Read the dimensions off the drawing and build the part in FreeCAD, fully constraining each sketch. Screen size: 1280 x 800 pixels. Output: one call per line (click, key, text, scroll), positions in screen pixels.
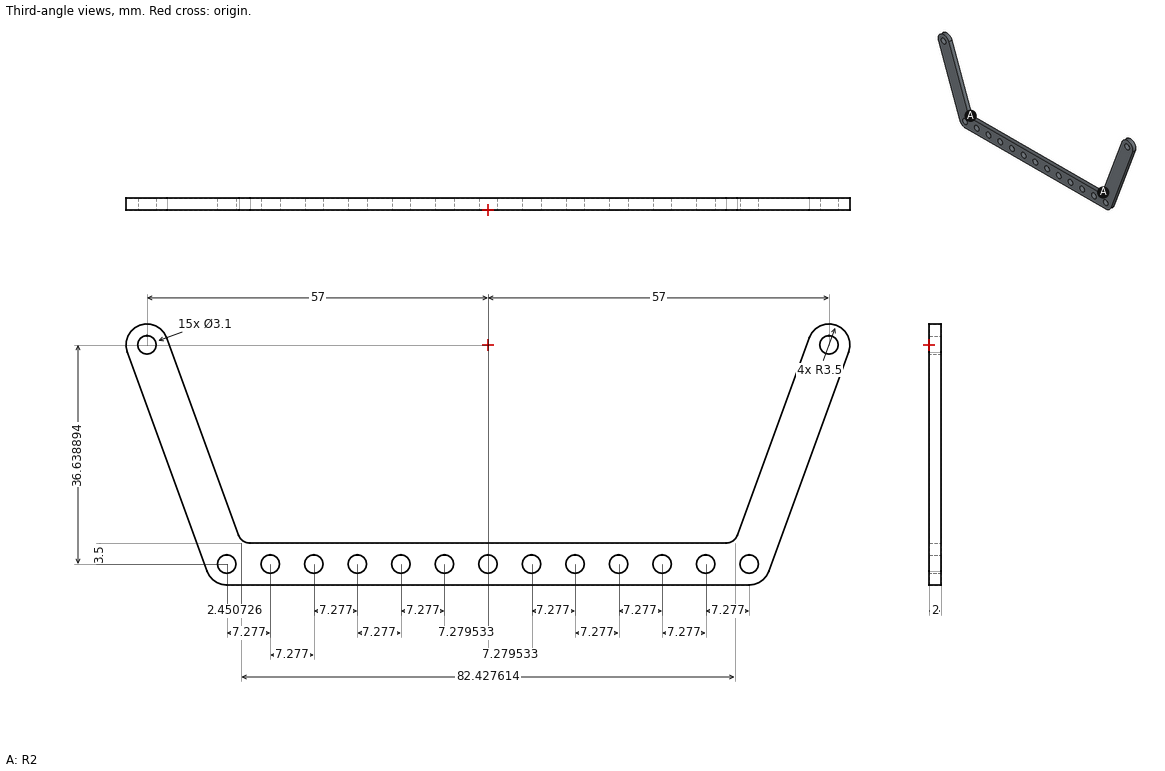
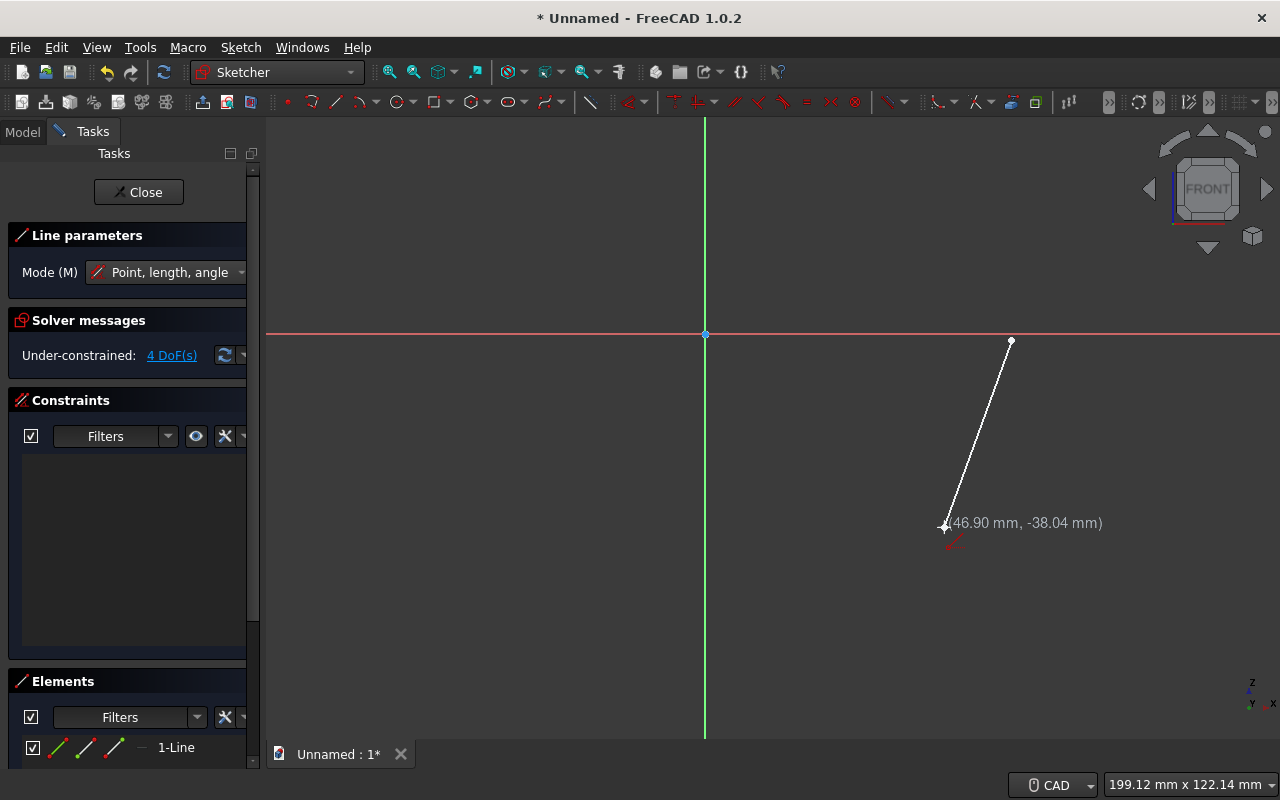
click(927, 539)
click(483, 539)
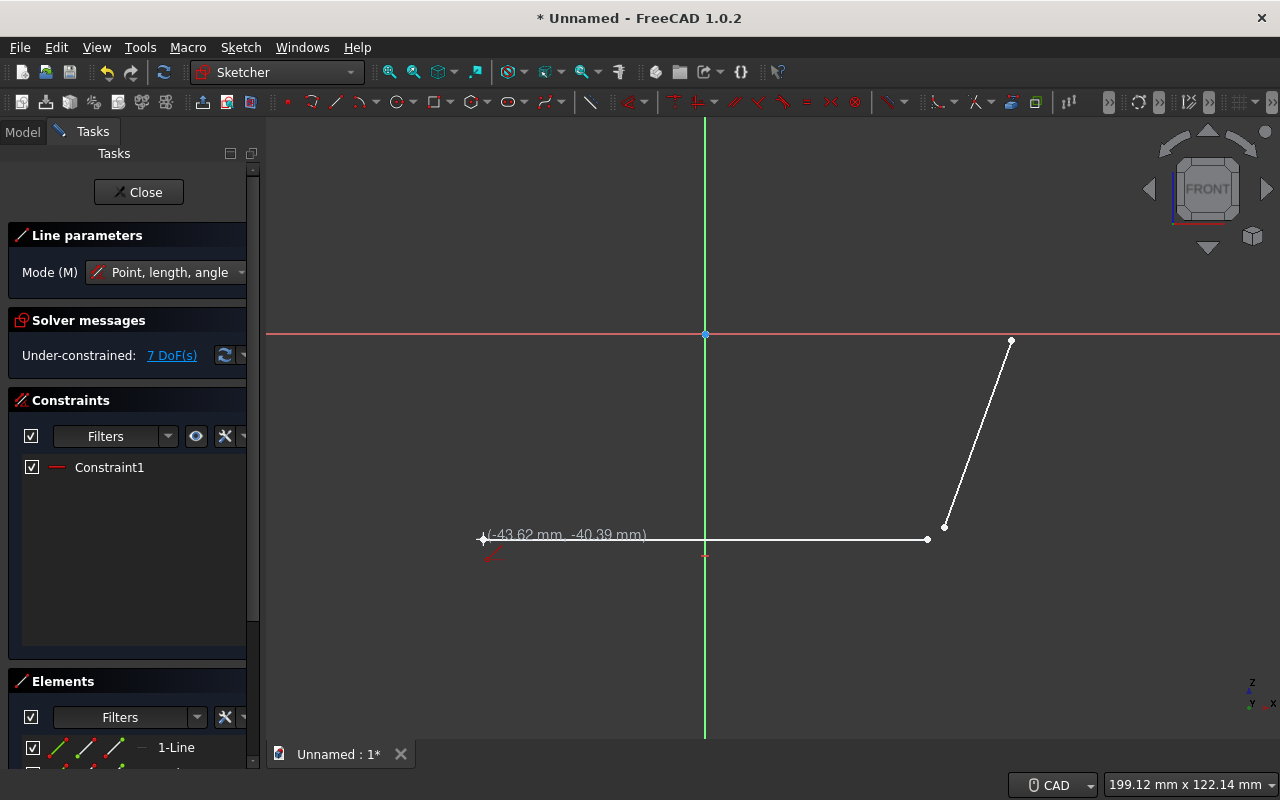
click(466, 527)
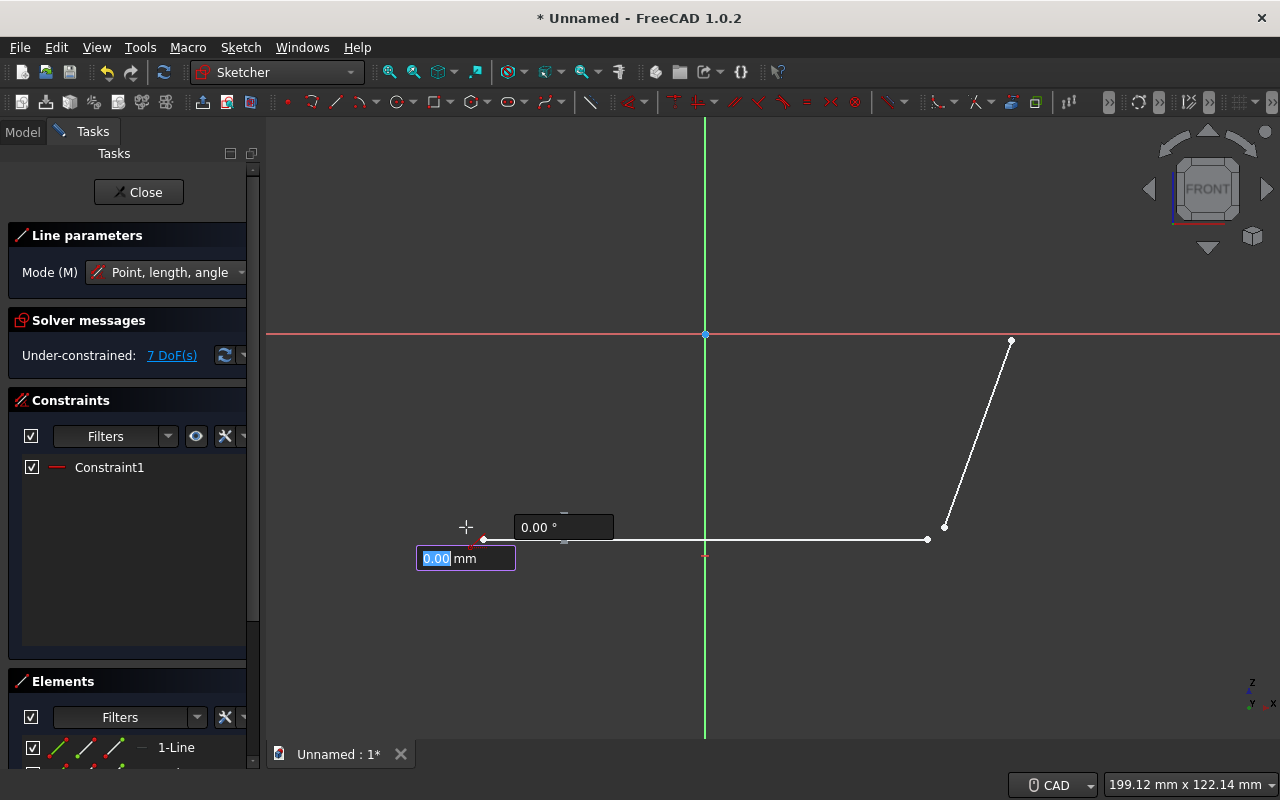
scroll(398, 340, up, 5)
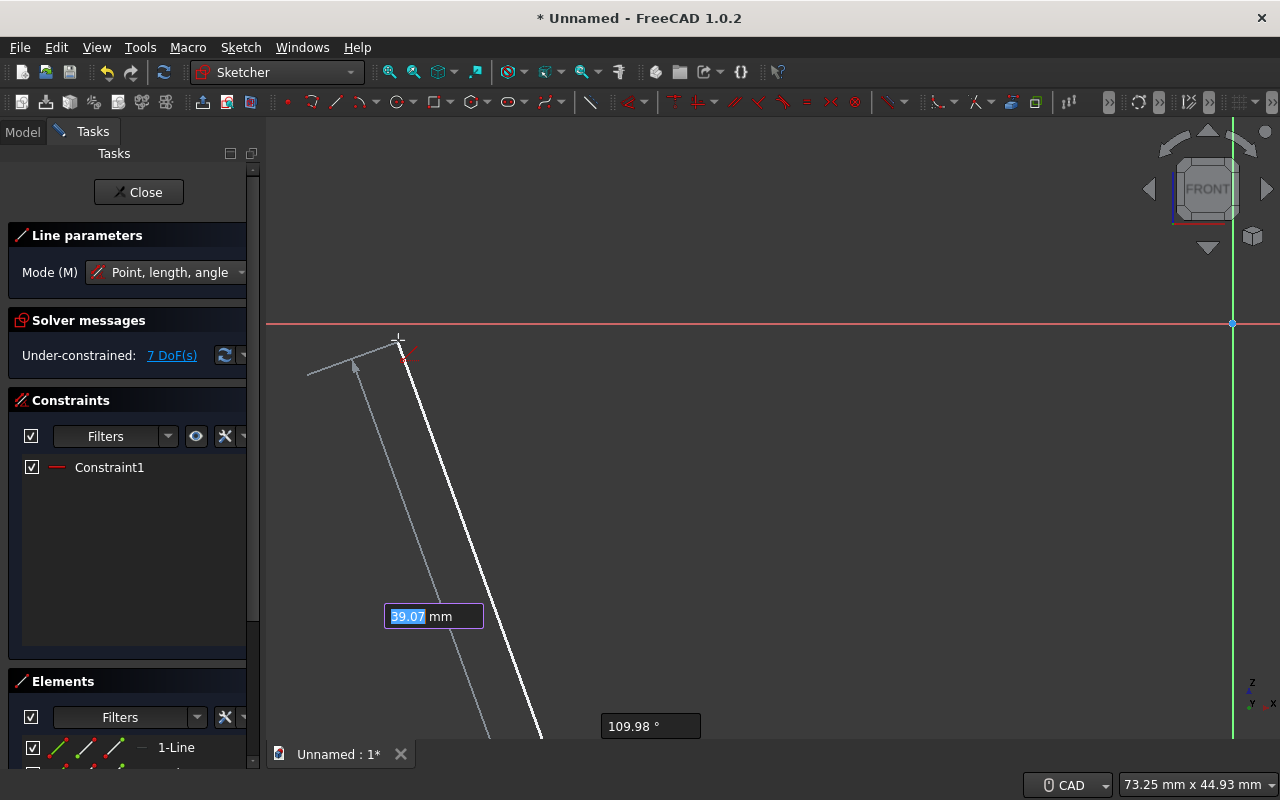
click(398, 340)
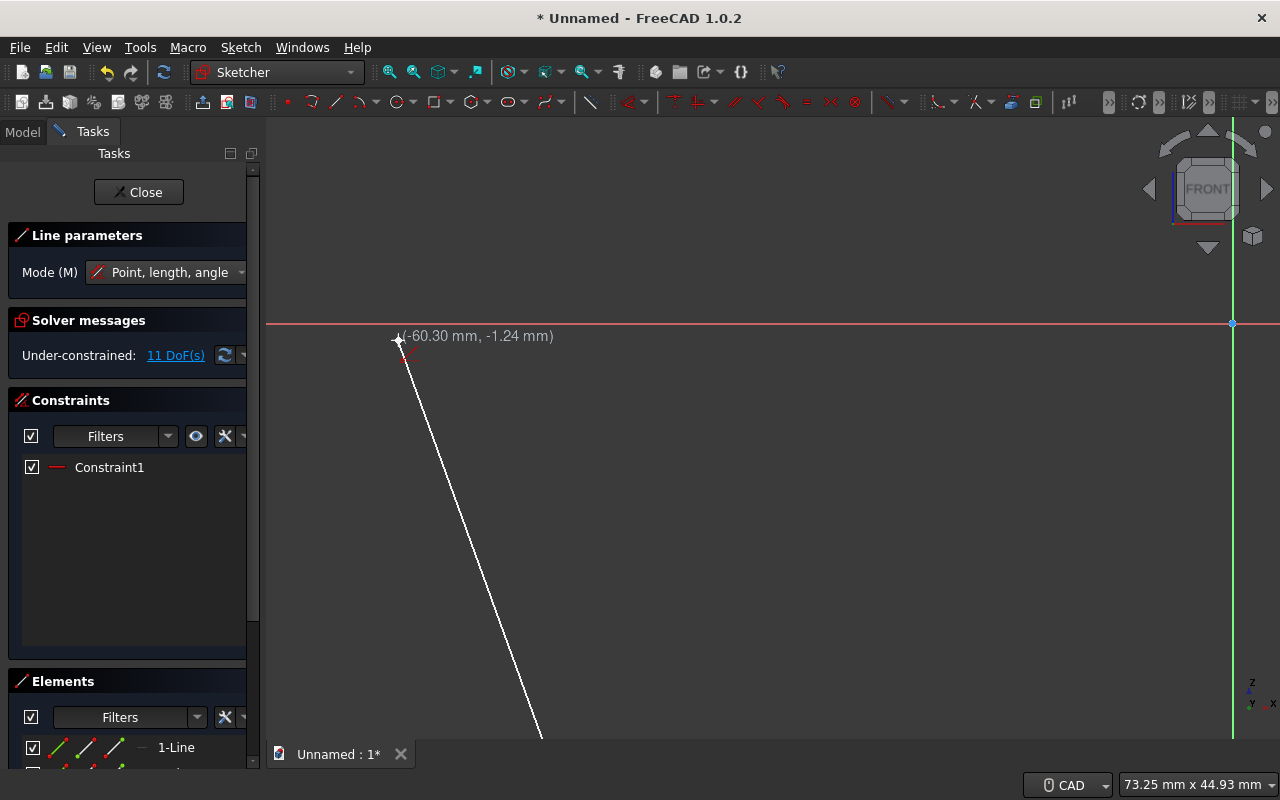
key(g)
key(m)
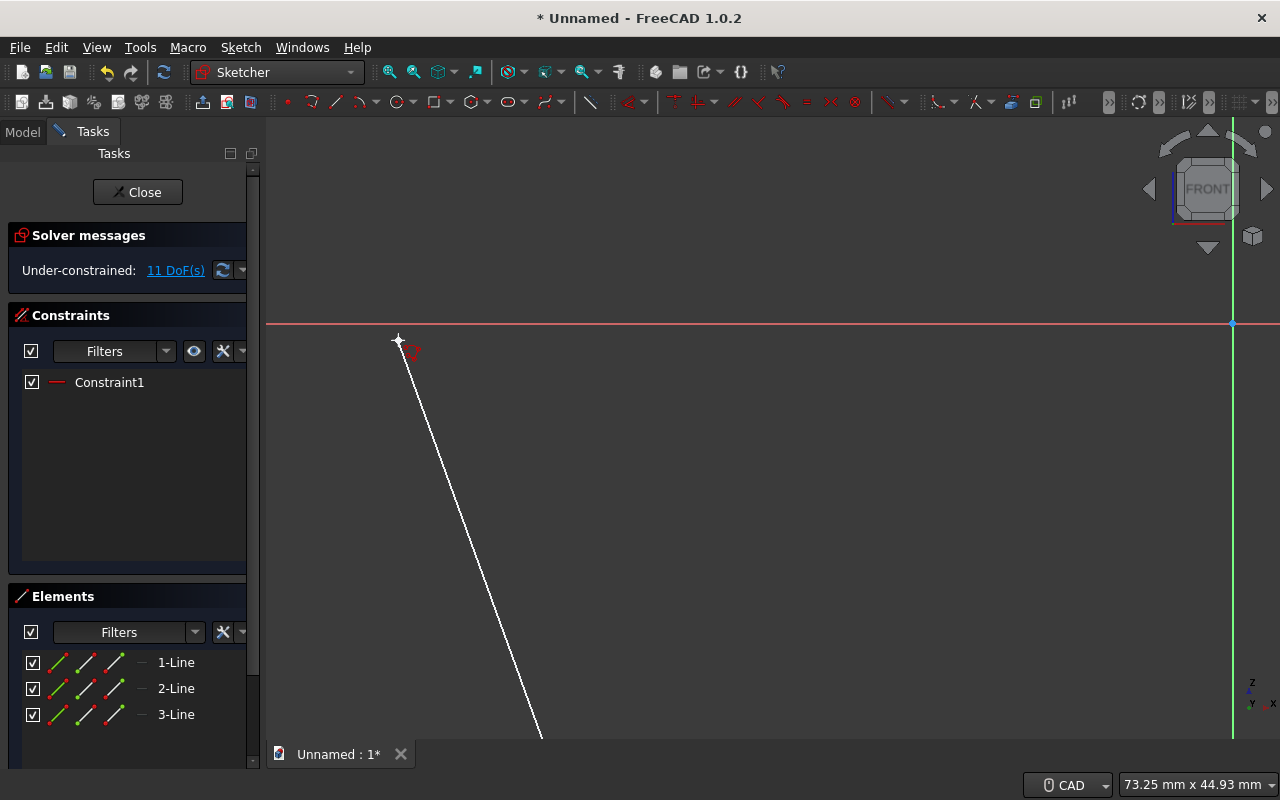
click(489, 307)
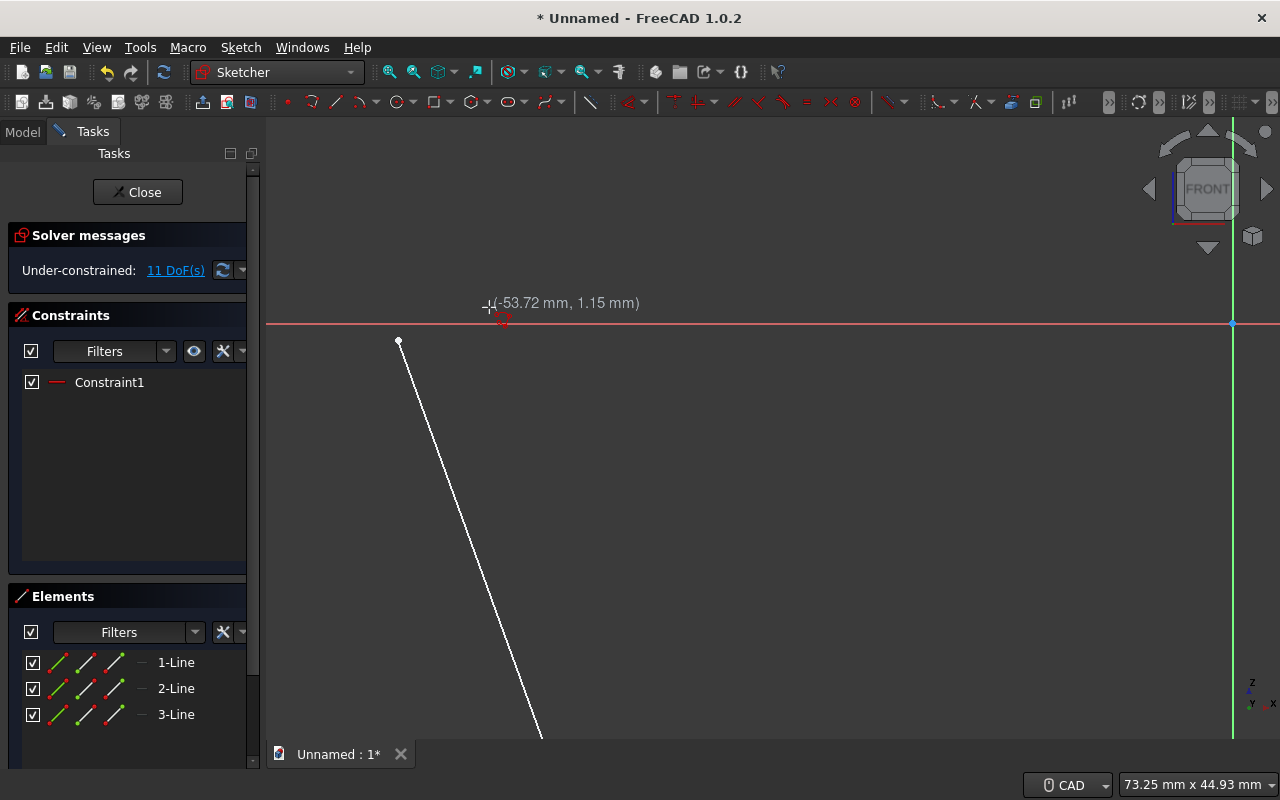
scroll(397, 340, down, 5)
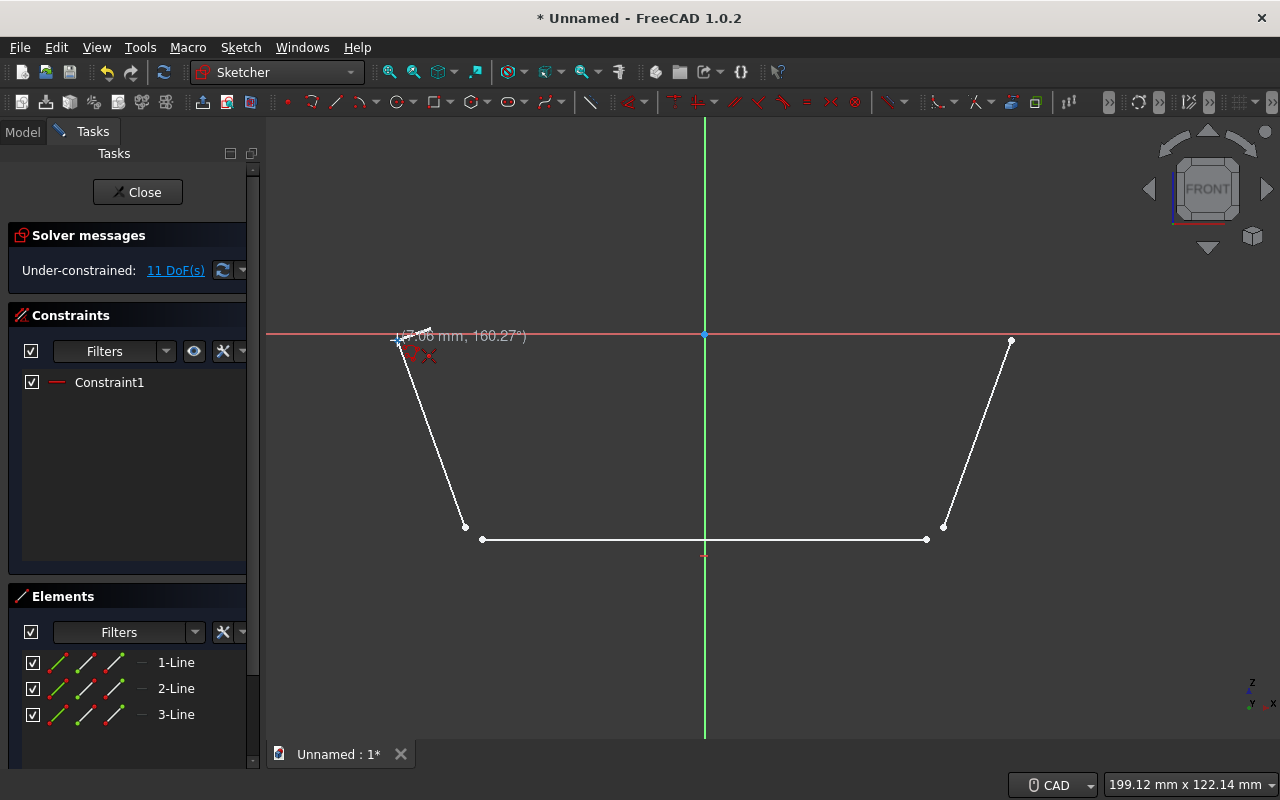
click(495, 503)
click(914, 503)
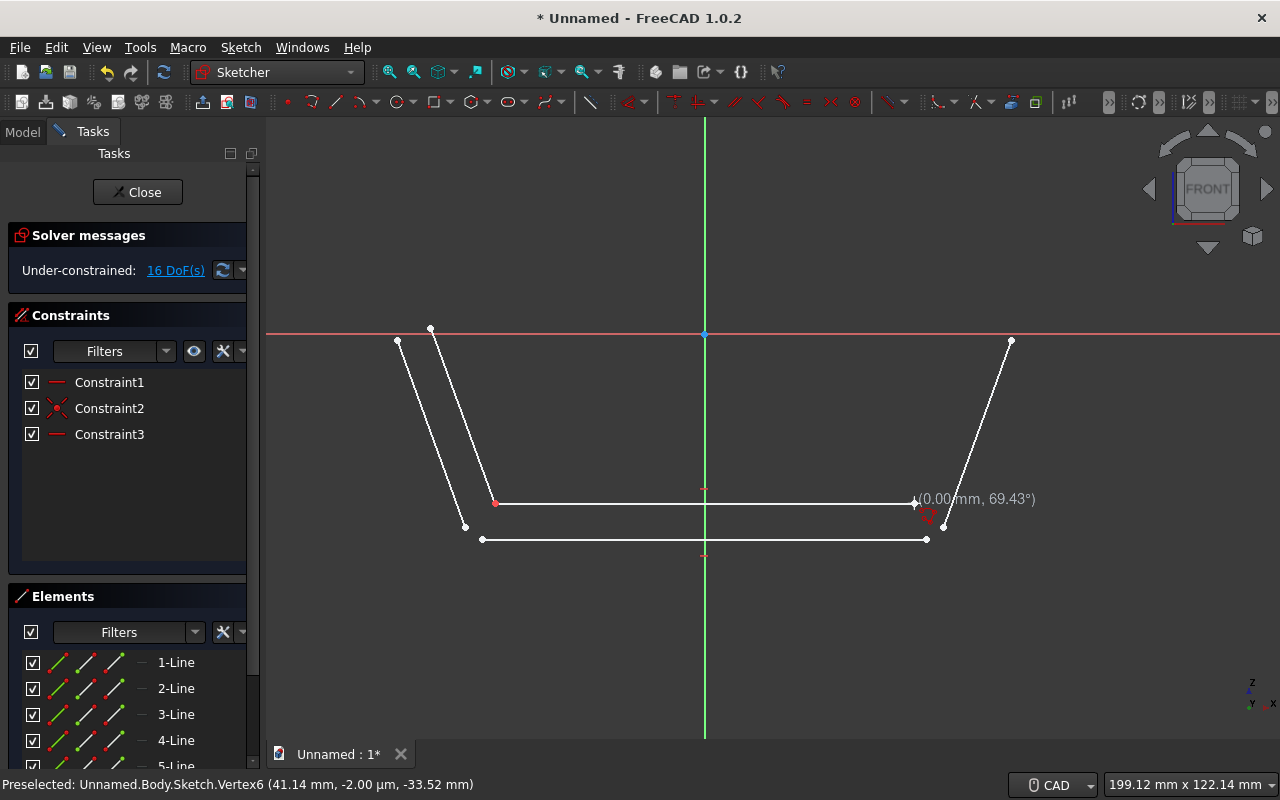
scroll(978, 328, up, 5)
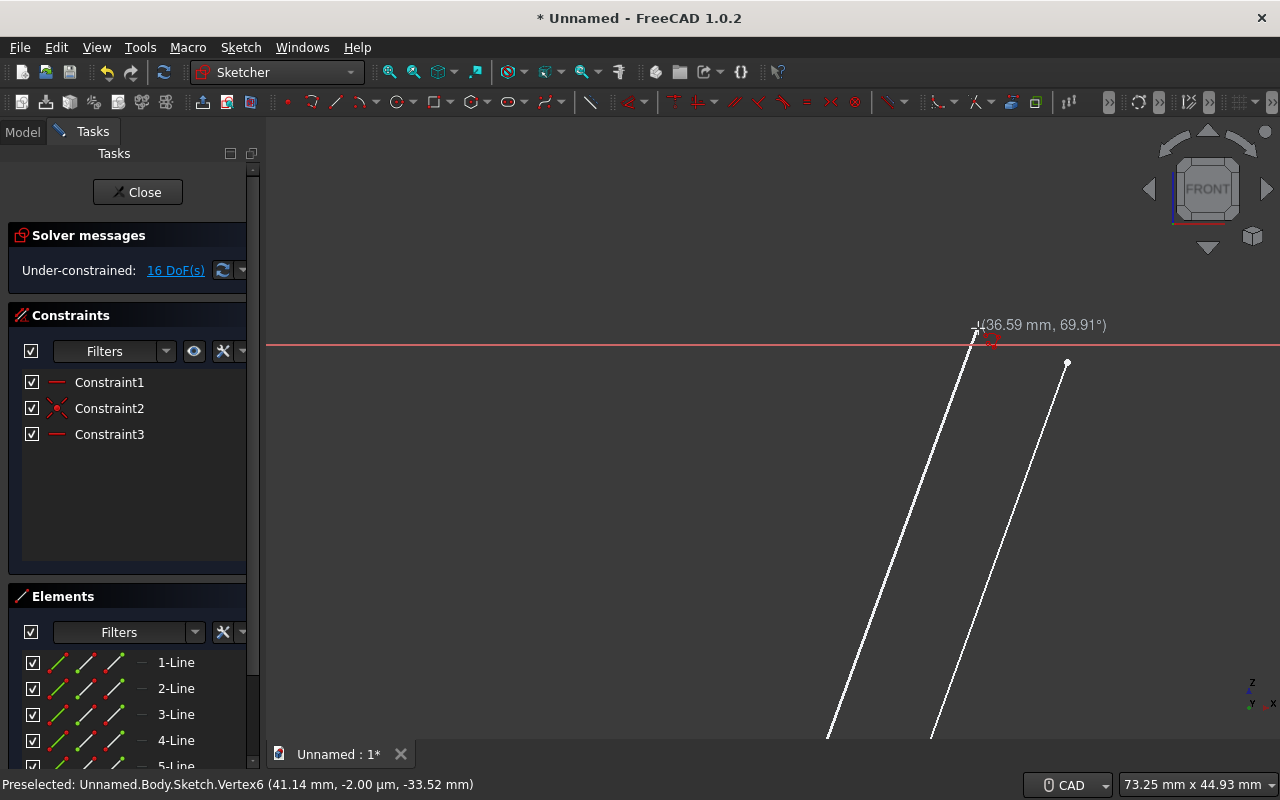
click(977, 328)
right_click(977, 328)